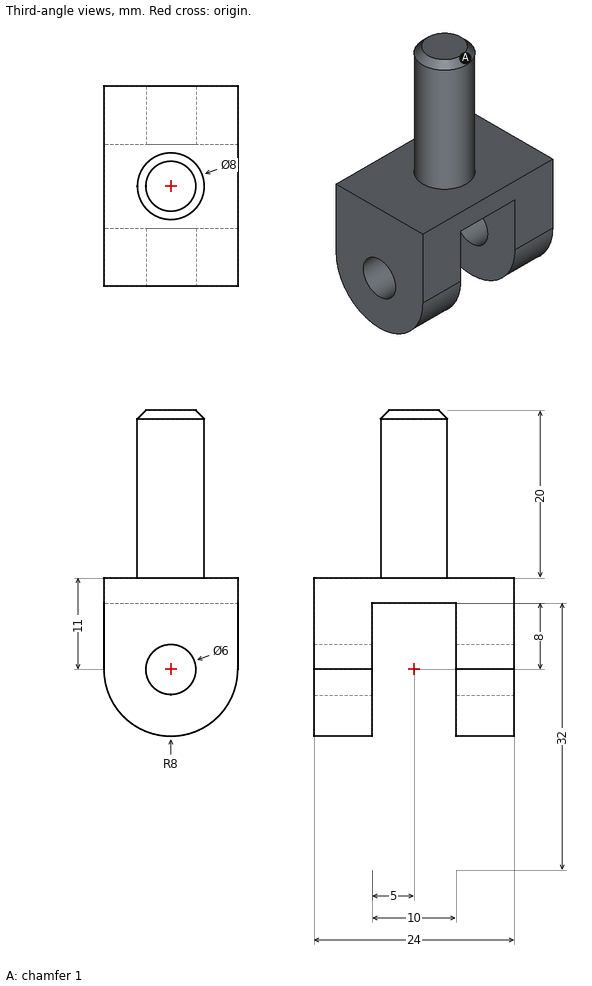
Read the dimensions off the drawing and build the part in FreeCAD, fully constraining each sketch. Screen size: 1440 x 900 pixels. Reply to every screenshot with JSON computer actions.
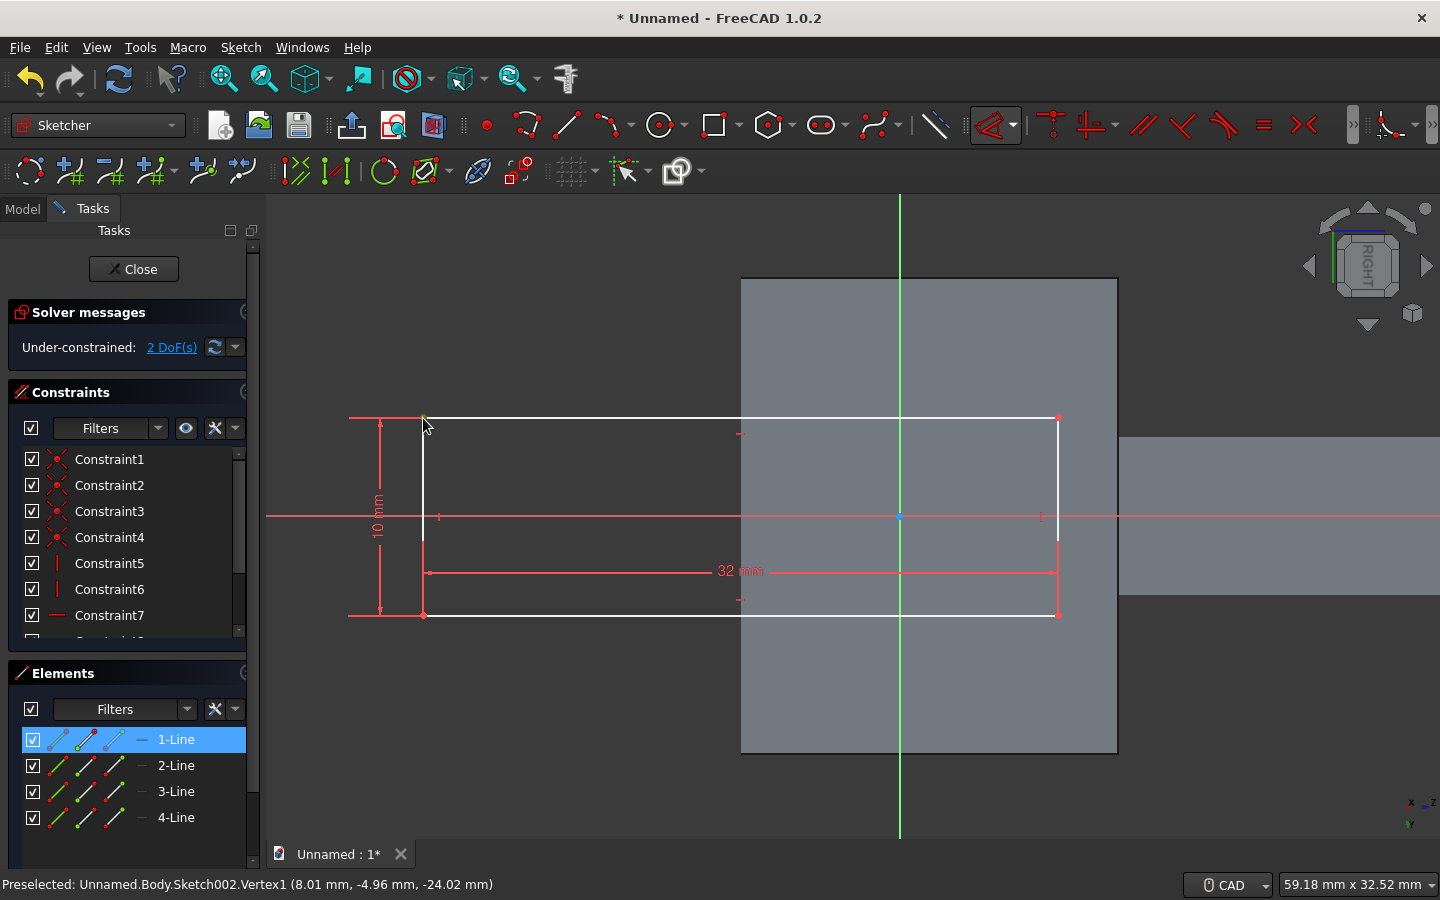
{"action": "key", "text": "i"}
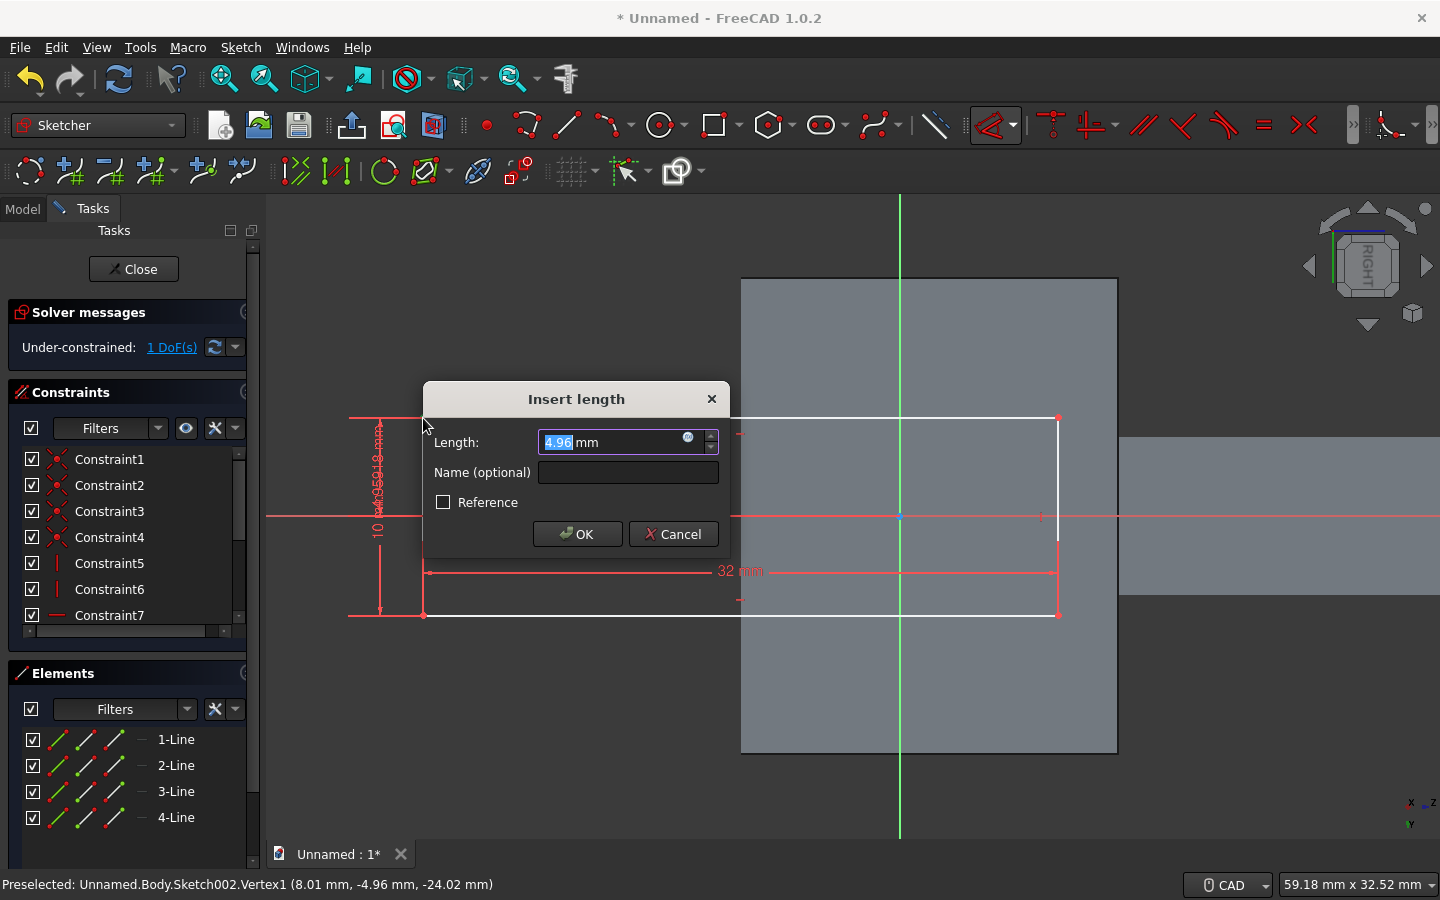
{"action": "type", "text": "5"}
{"action": "key", "text": "Return"}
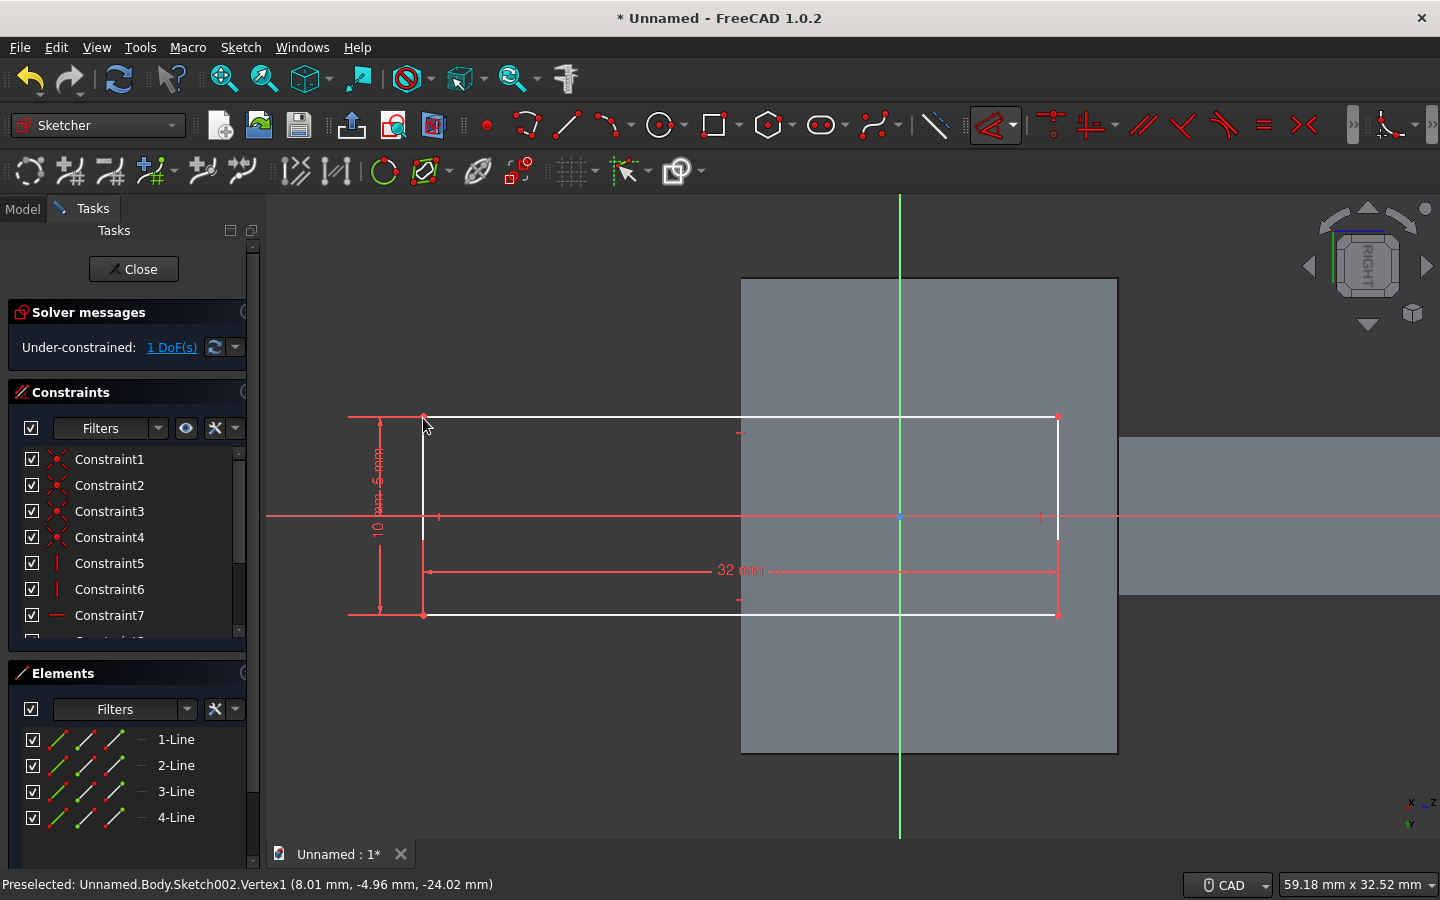
{"action": "left_click", "coordinate": [1058, 615]}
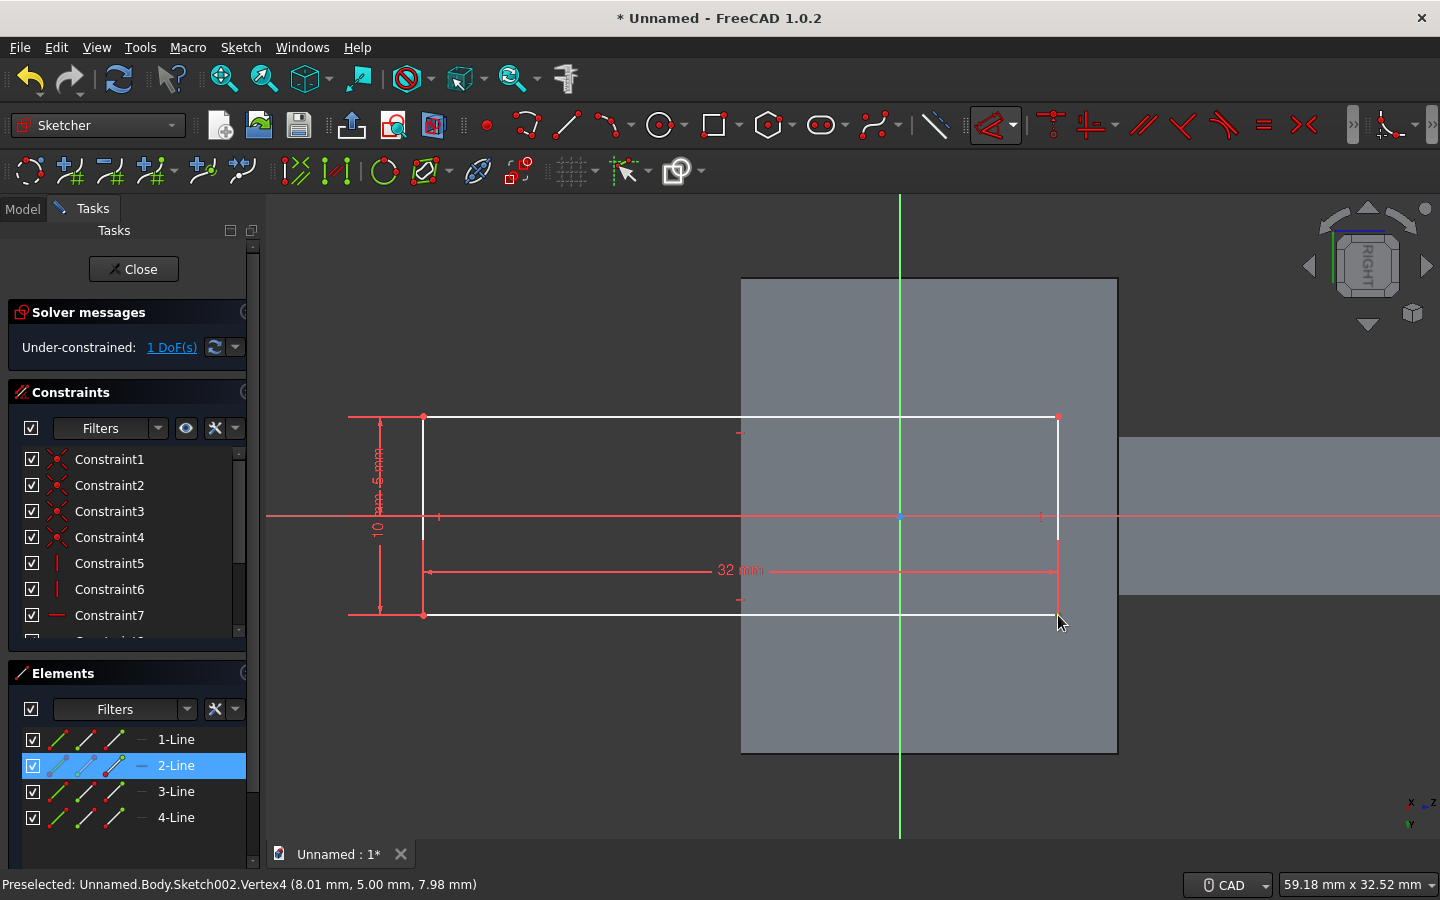
{"action": "key", "text": "l"}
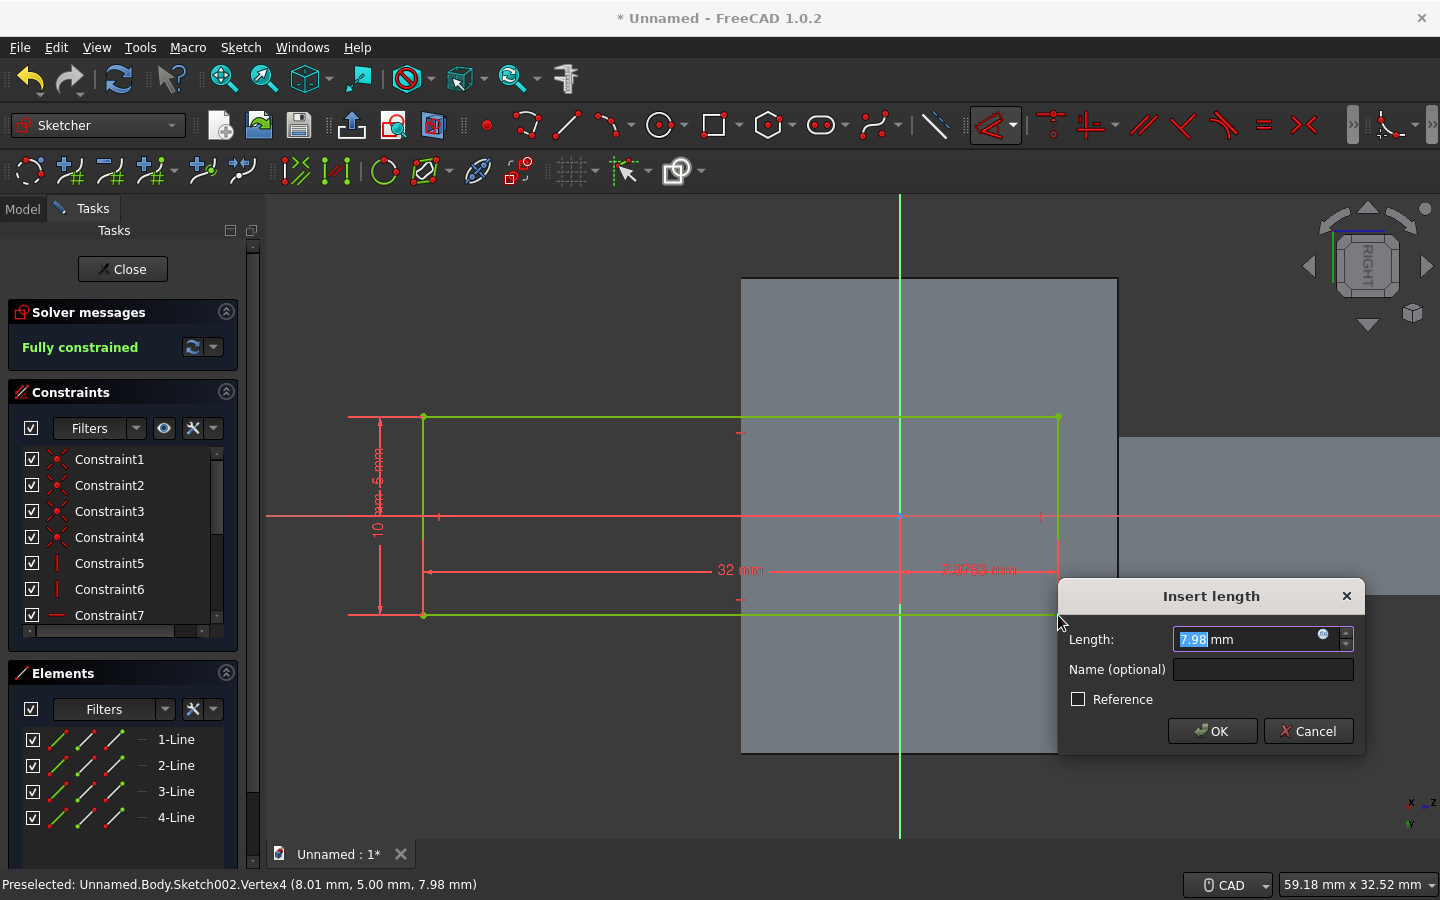
{"action": "type", "text": "8"}
{"action": "key", "text": "Return"}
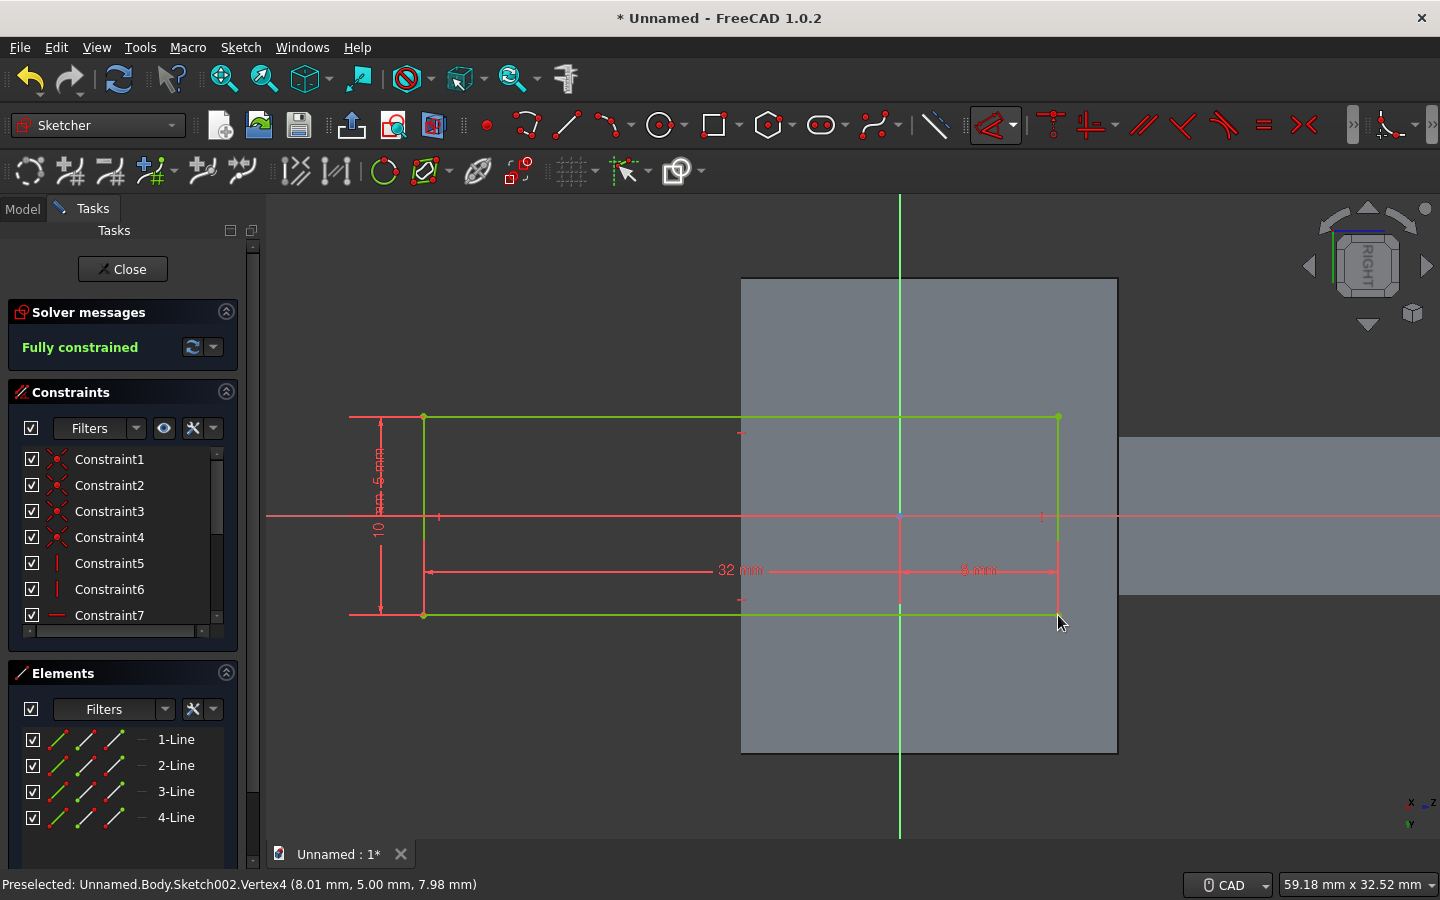
{"action": "left_click", "coordinate": [123, 269]}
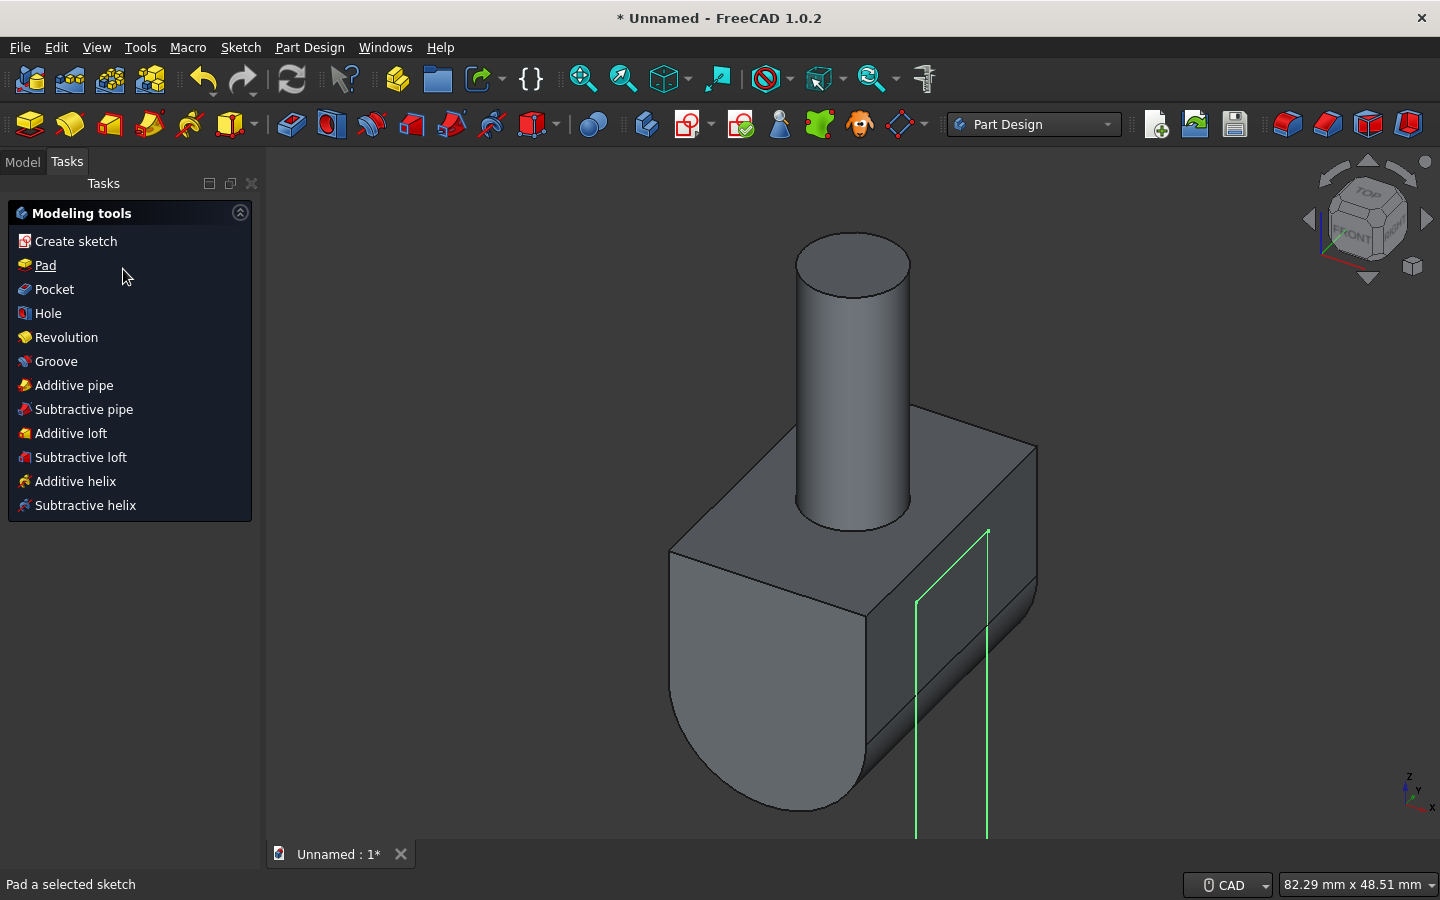
{"action": "left_click", "coordinate": [292, 124]}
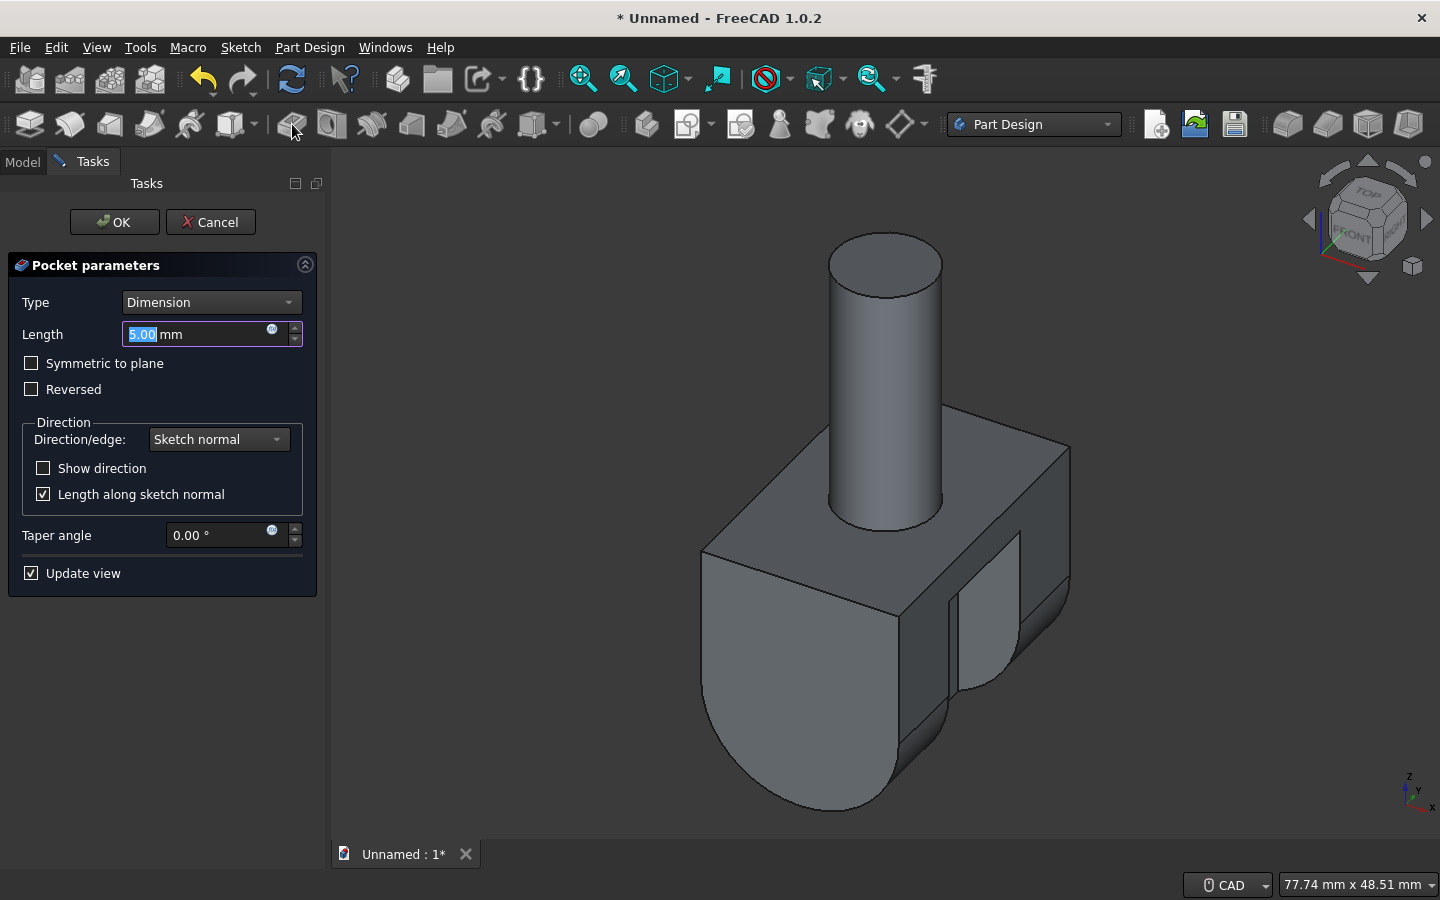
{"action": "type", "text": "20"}
{"action": "key", "text": "Tab"}